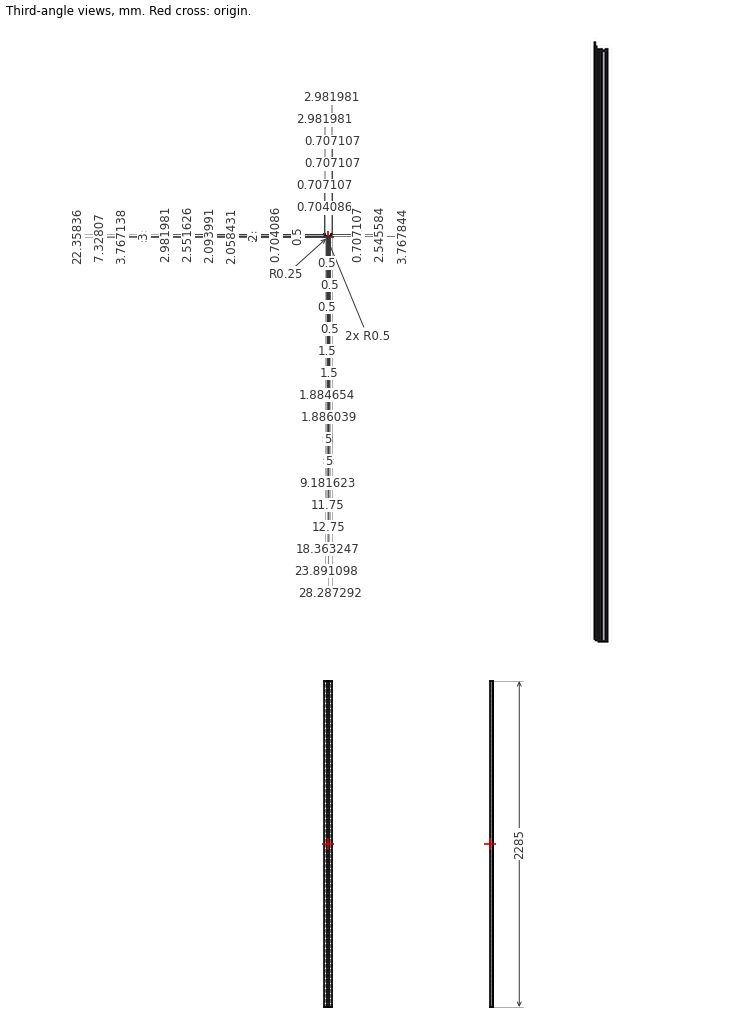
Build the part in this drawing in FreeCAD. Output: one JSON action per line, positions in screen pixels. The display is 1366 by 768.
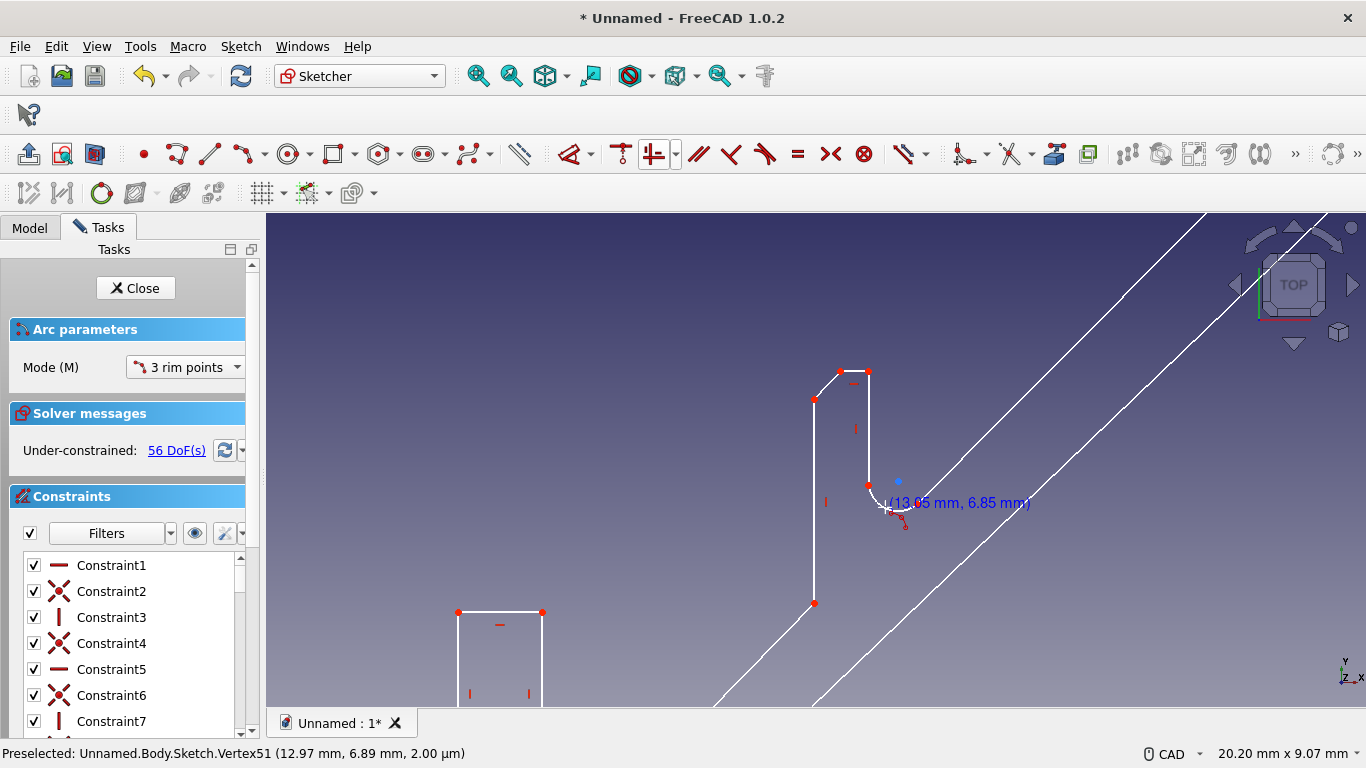
{"action": "scroll", "coordinate": [892, 508], "scroll_direction": "down", "scroll_amount": 8}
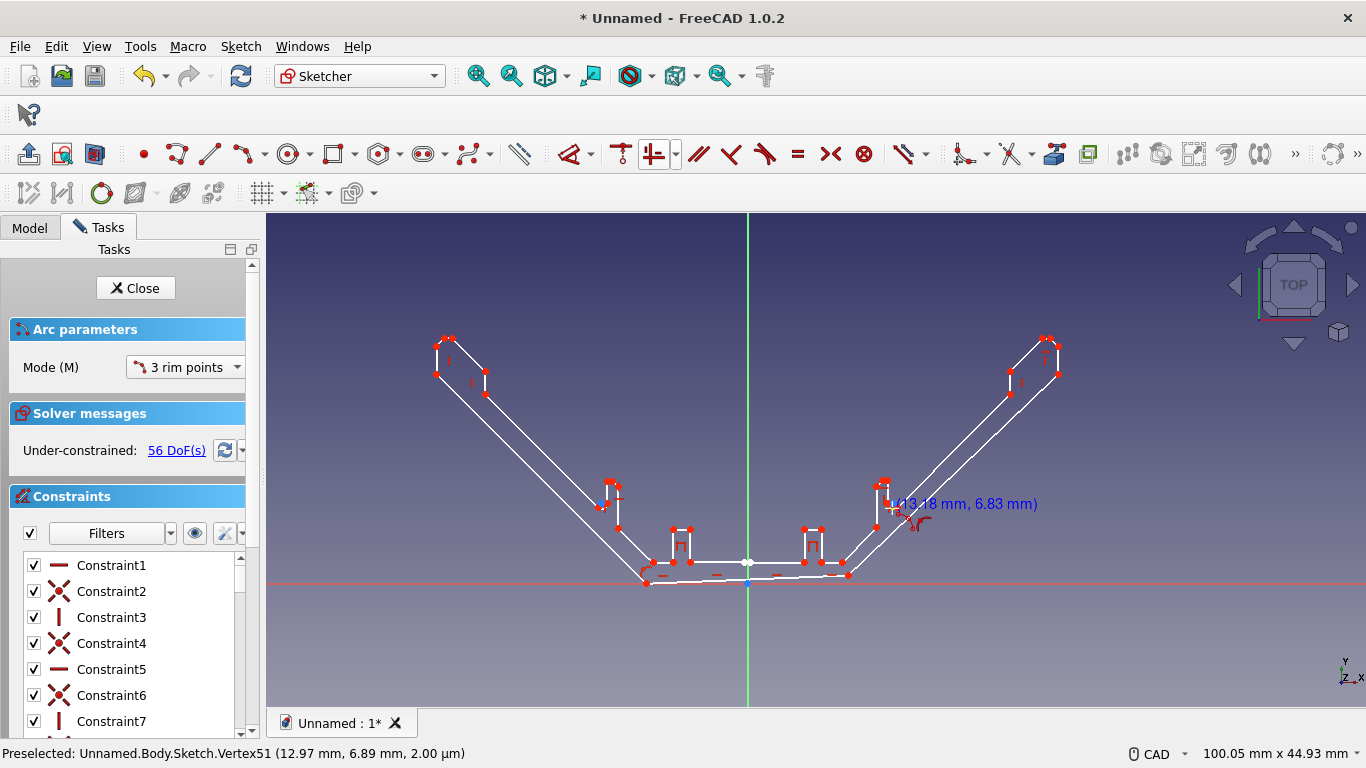
{"action": "scroll", "coordinate": [750, 562], "scroll_direction": "up", "scroll_amount": 9}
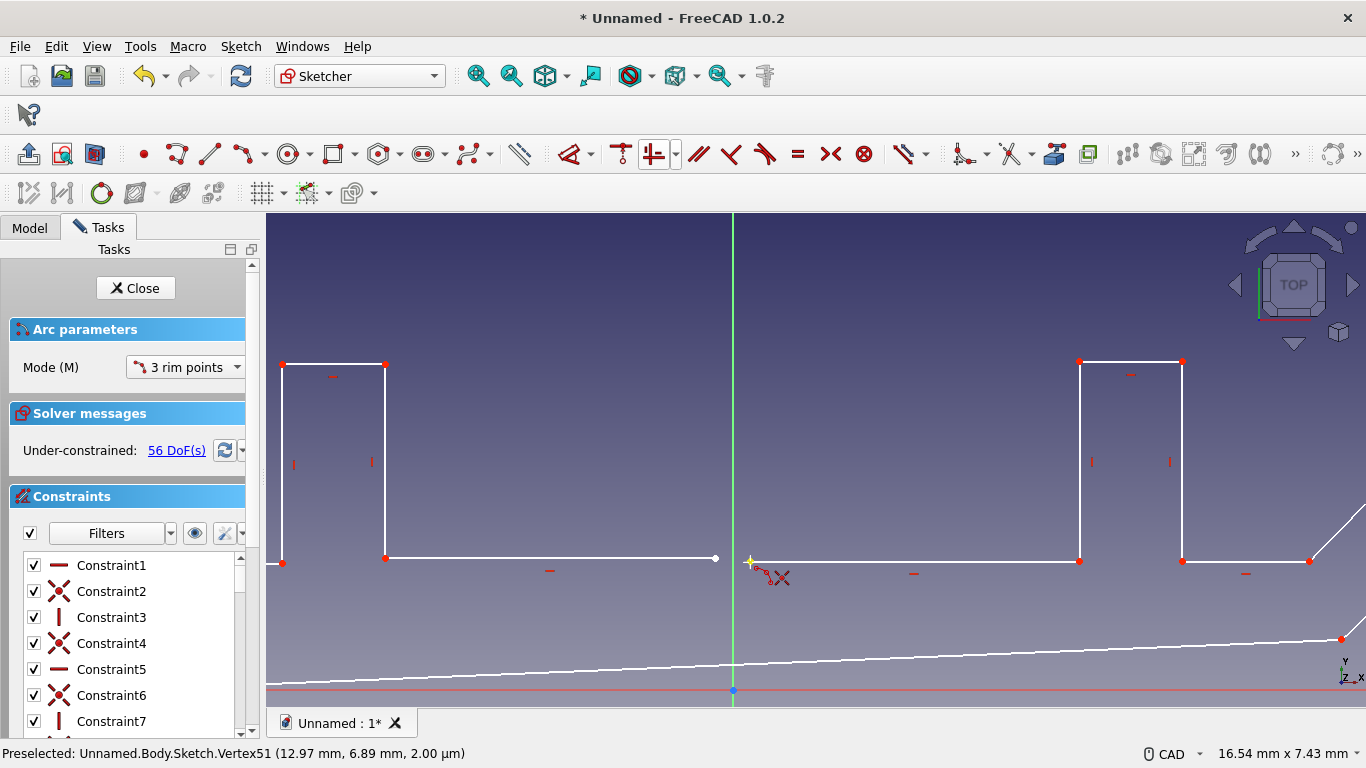
{"action": "left_click", "coordinate": [750, 562]}
{"action": "left_click", "coordinate": [716, 558]}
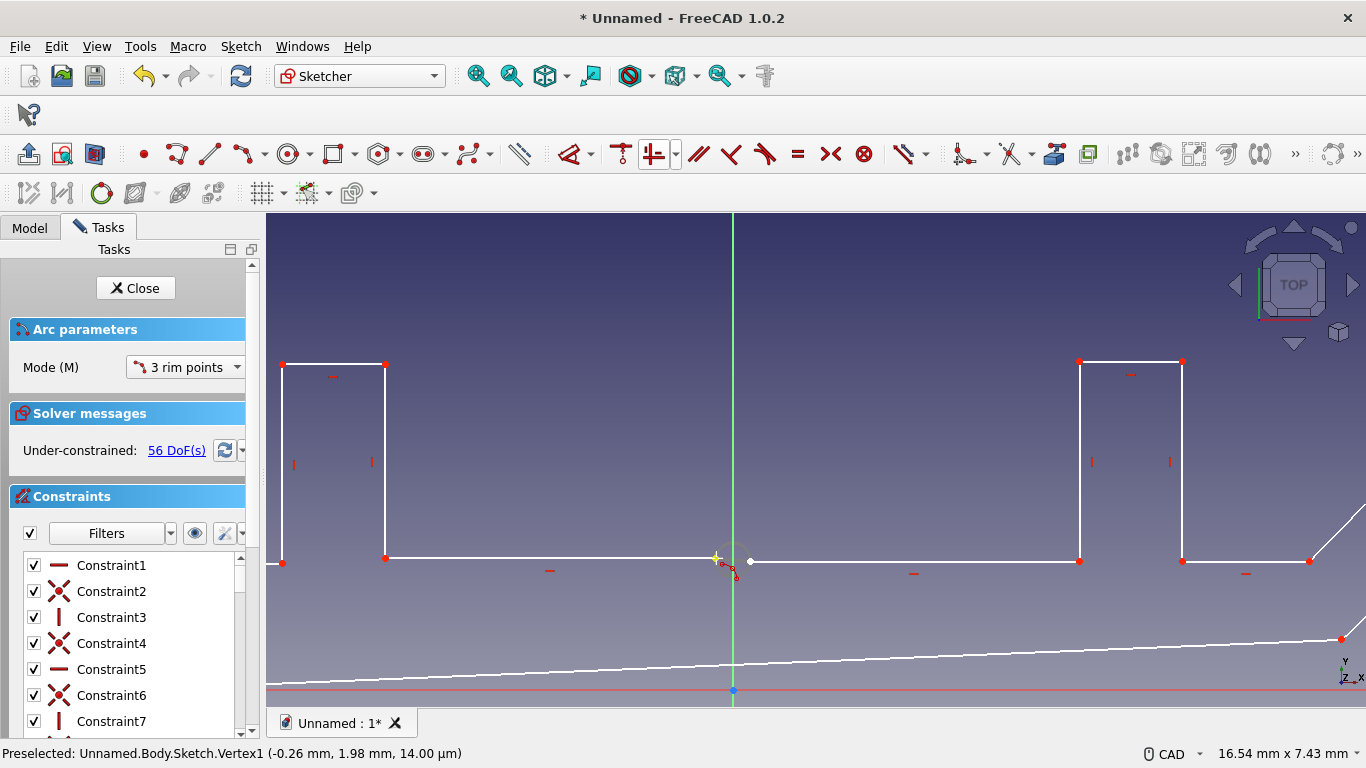
{"action": "scroll", "coordinate": [723, 571], "scroll_direction": "up", "scroll_amount": 3}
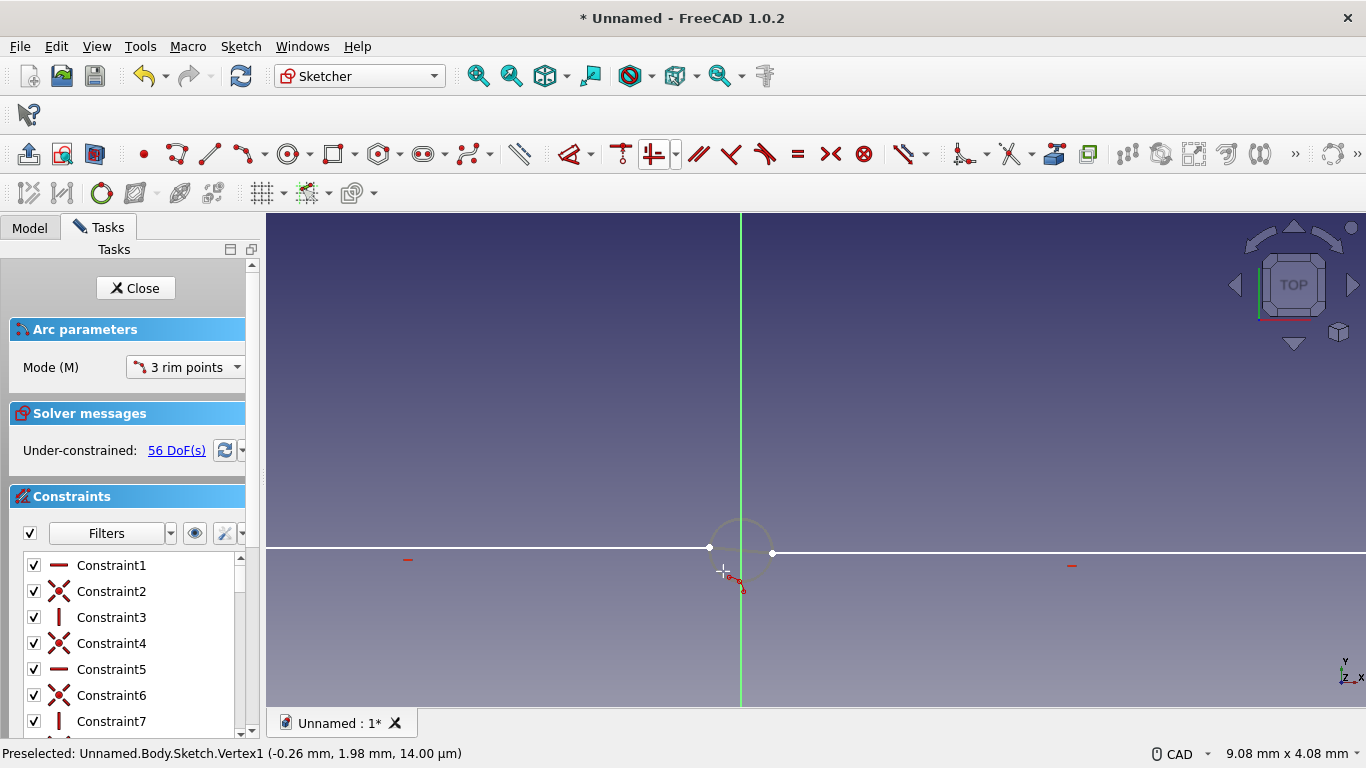
{"action": "left_click", "coordinate": [723, 570]}
{"action": "key", "text": "Escape"}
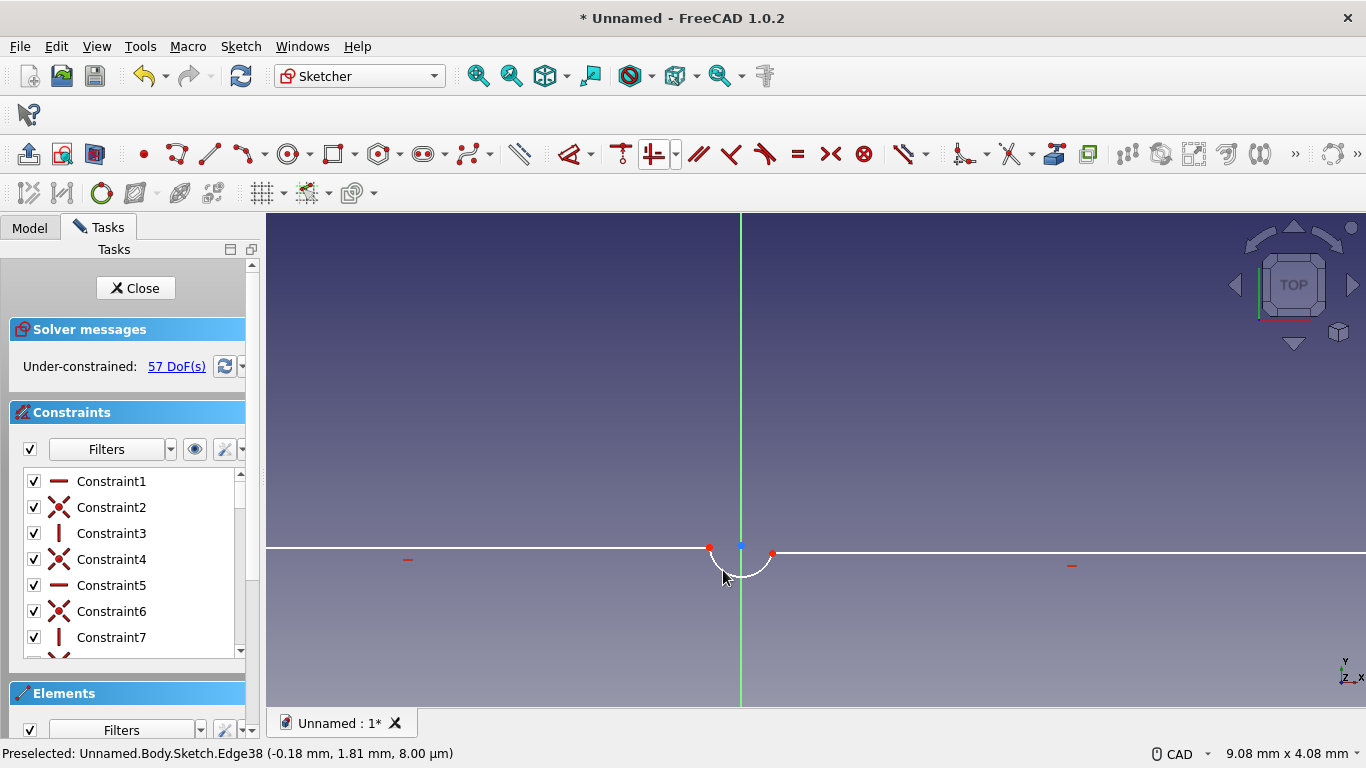
{"action": "scroll", "coordinate": [748, 562], "scroll_direction": "down", "scroll_amount": 12}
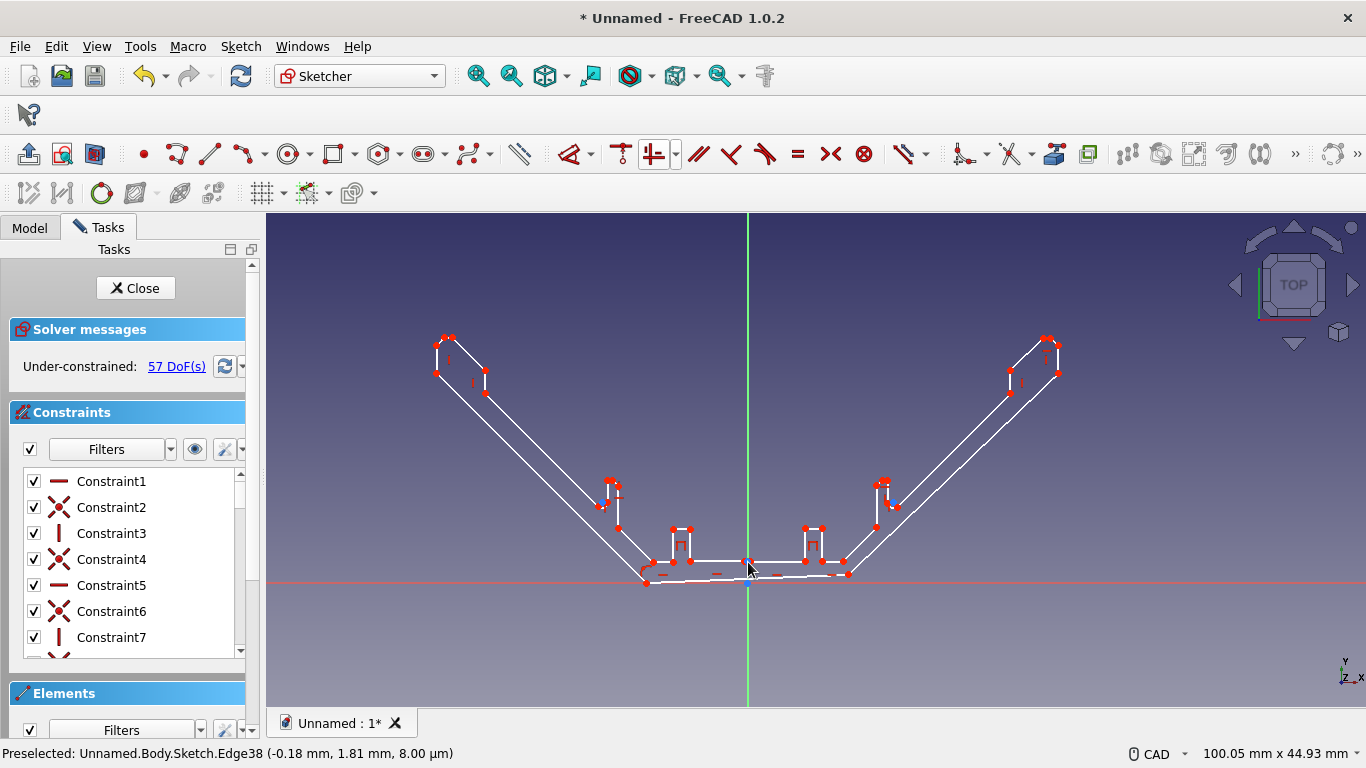
{"action": "scroll", "coordinate": [608, 487], "scroll_direction": "up", "scroll_amount": 4}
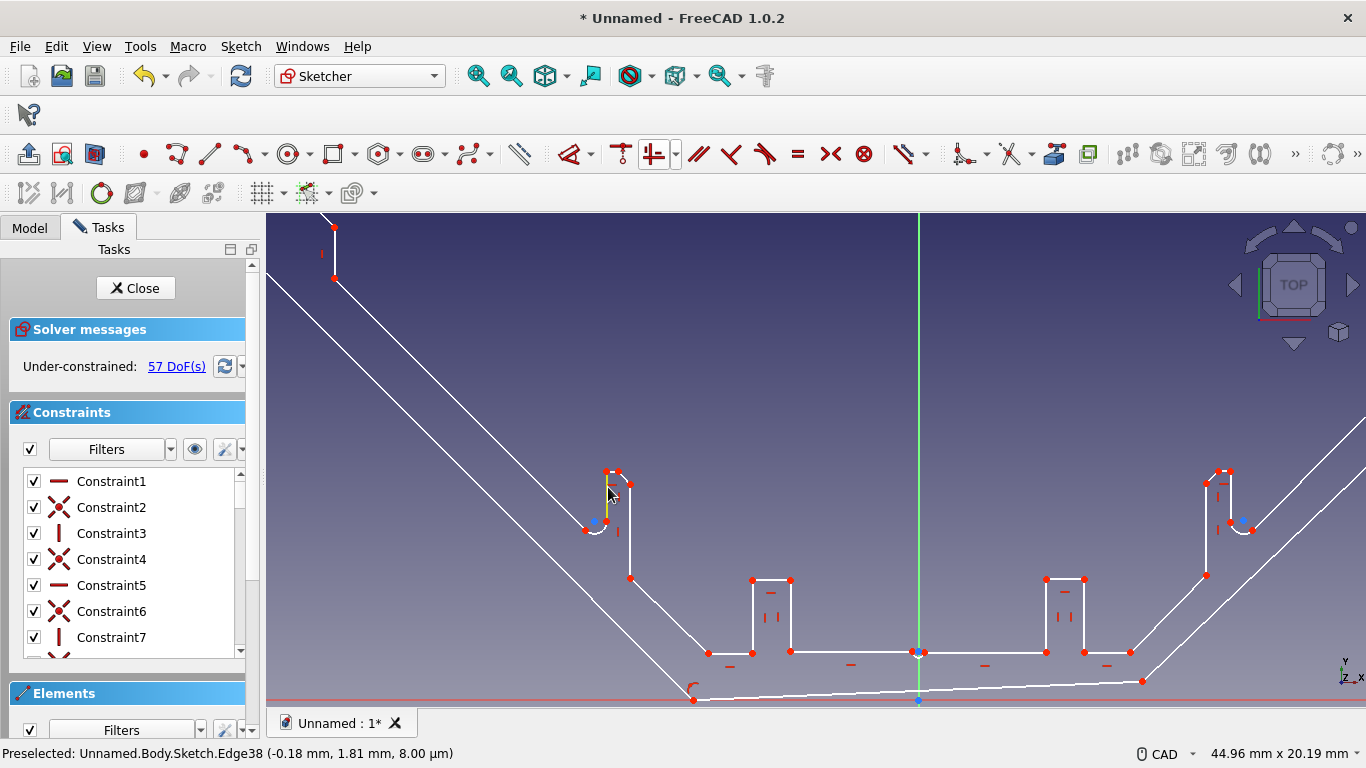
{"action": "left_click", "coordinate": [607, 507]}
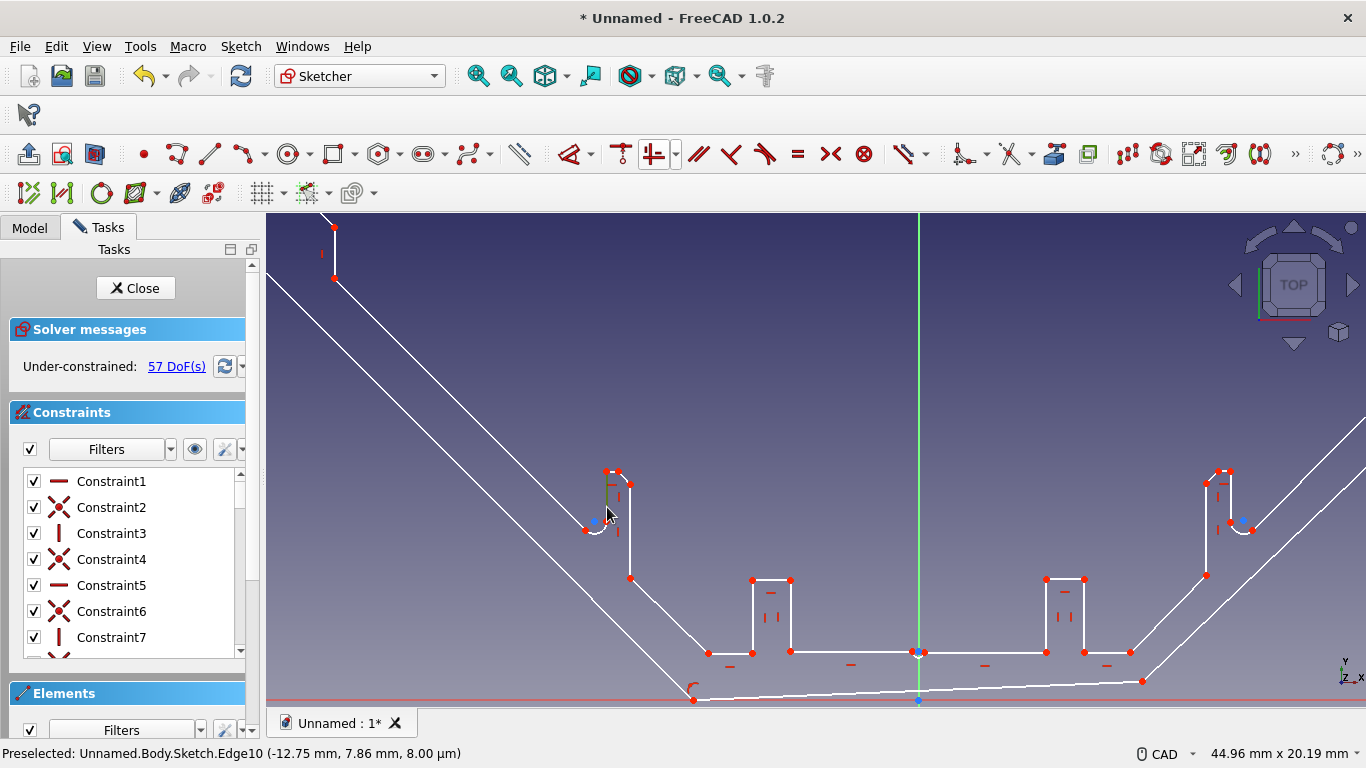
{"action": "left_click", "coordinate": [599, 533]}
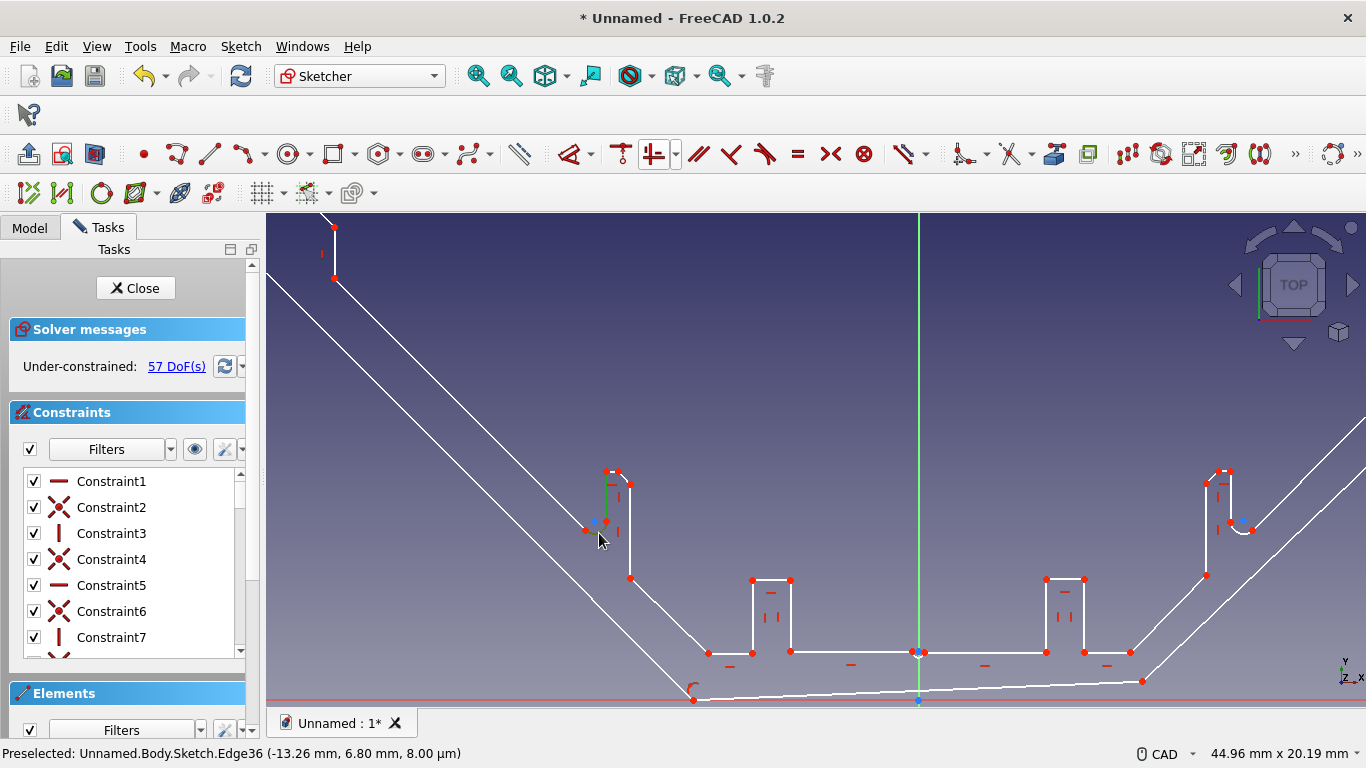
{"action": "left_click", "coordinate": [765, 154]}